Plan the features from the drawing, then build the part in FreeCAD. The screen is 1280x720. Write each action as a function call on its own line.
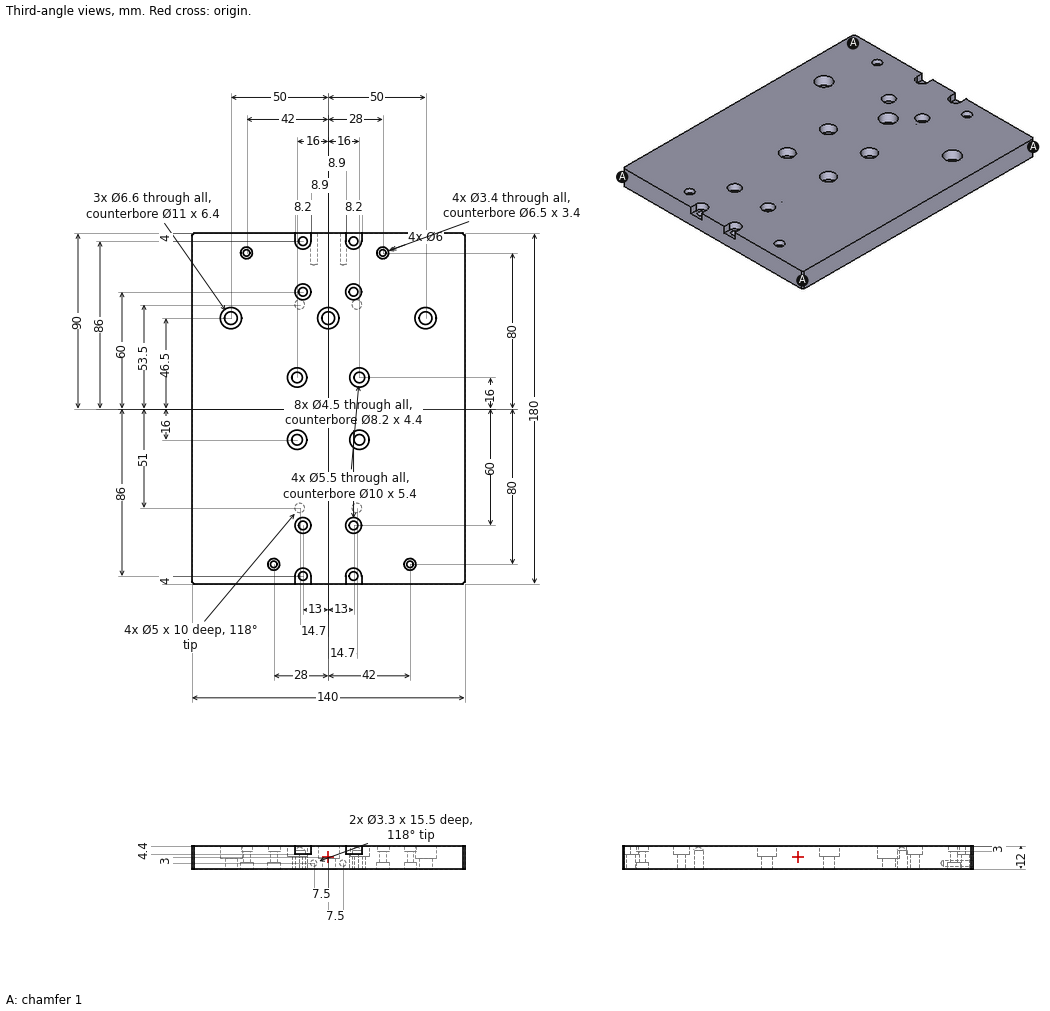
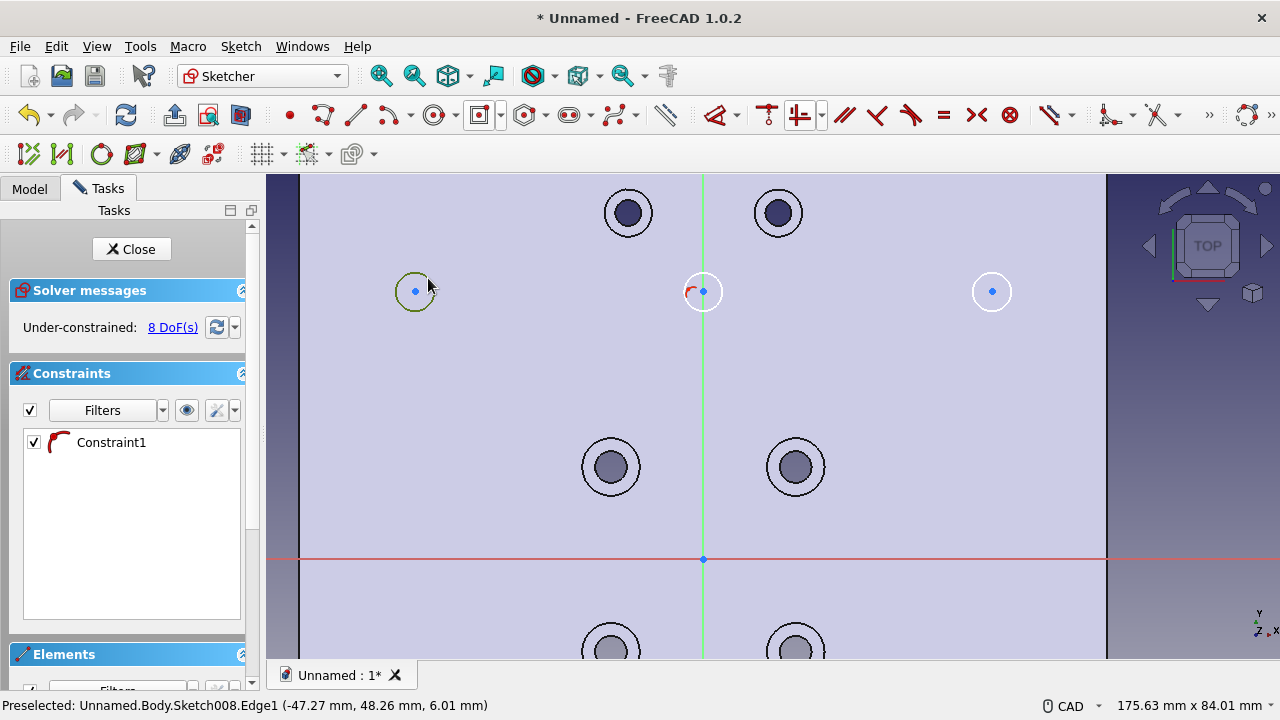
click(717, 279)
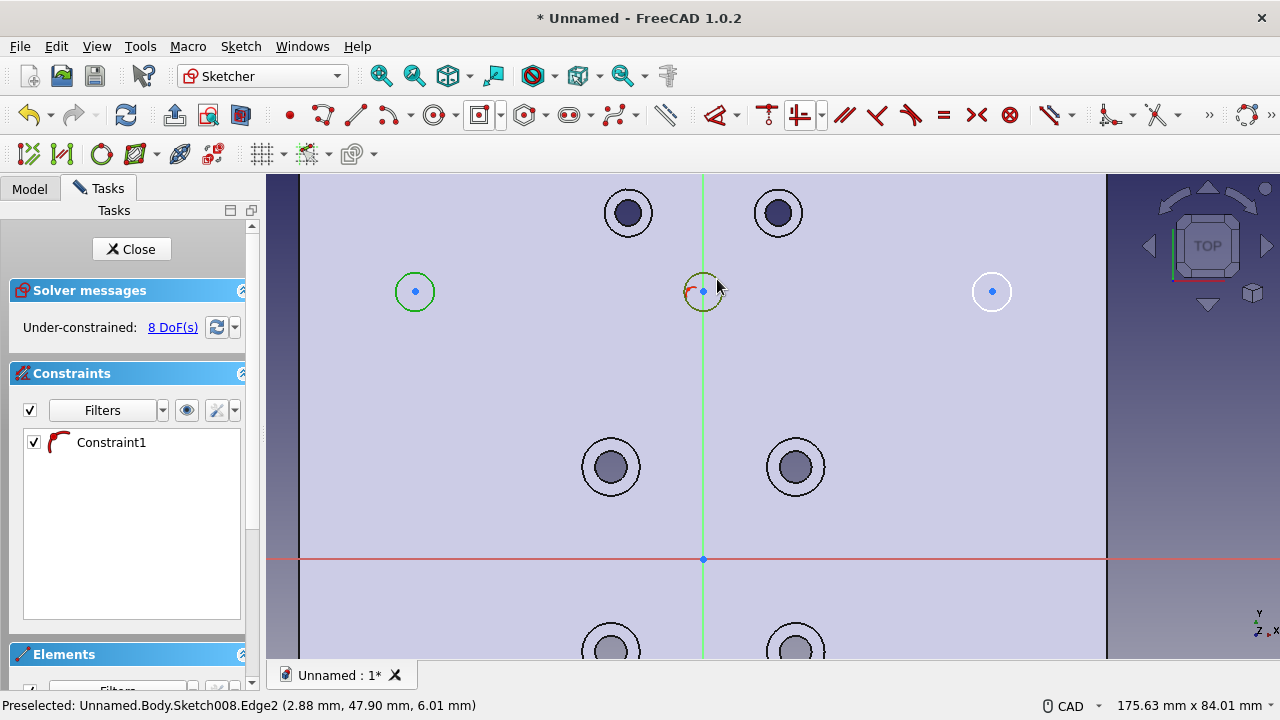
click(1005, 278)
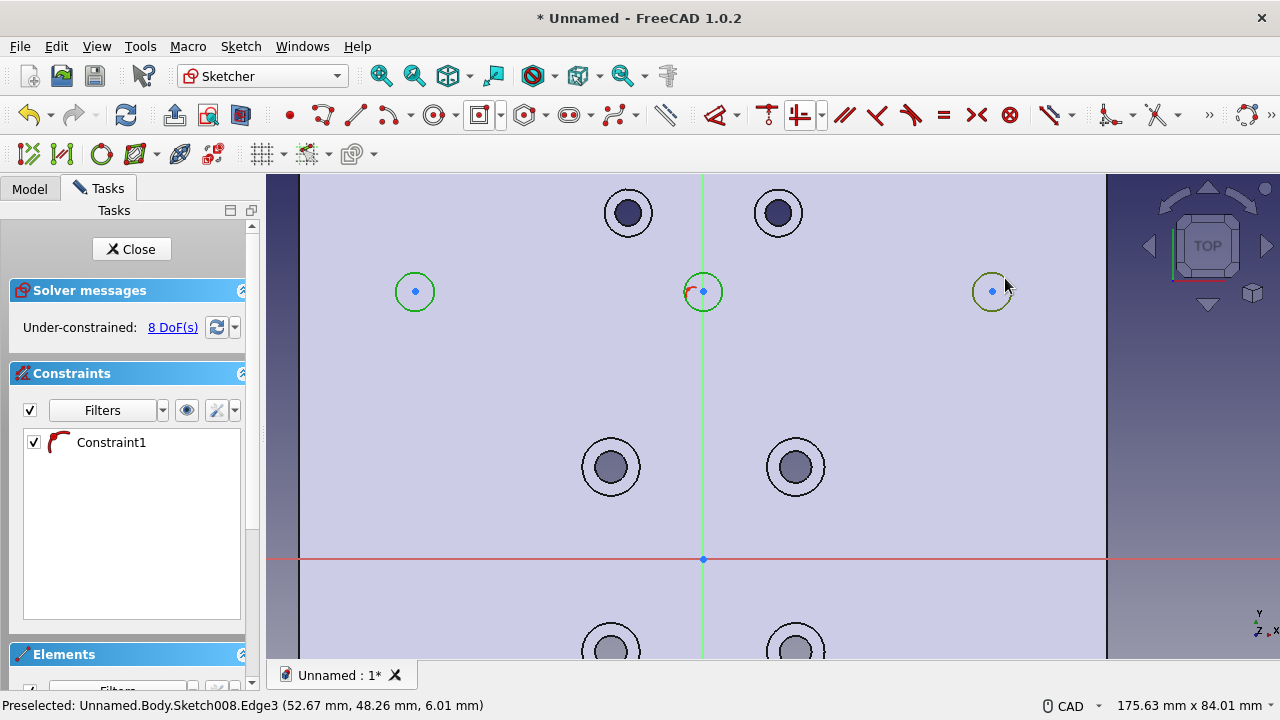
click(944, 116)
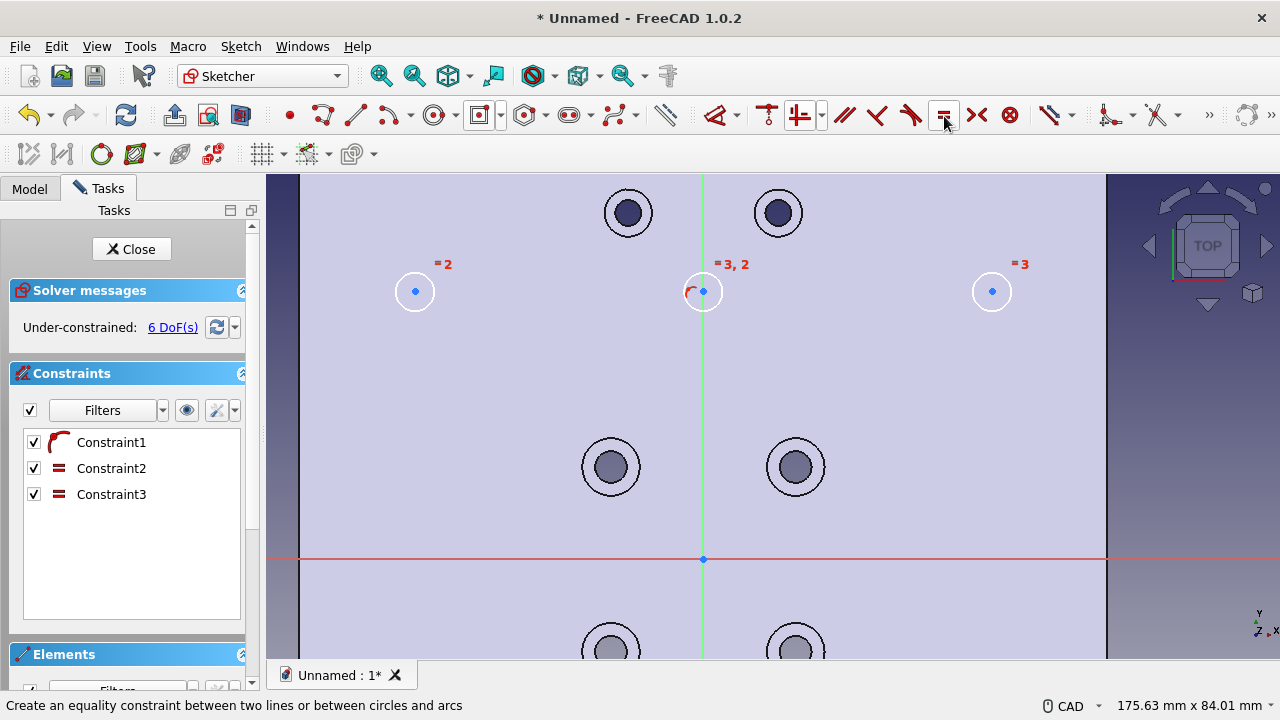
click(714, 116)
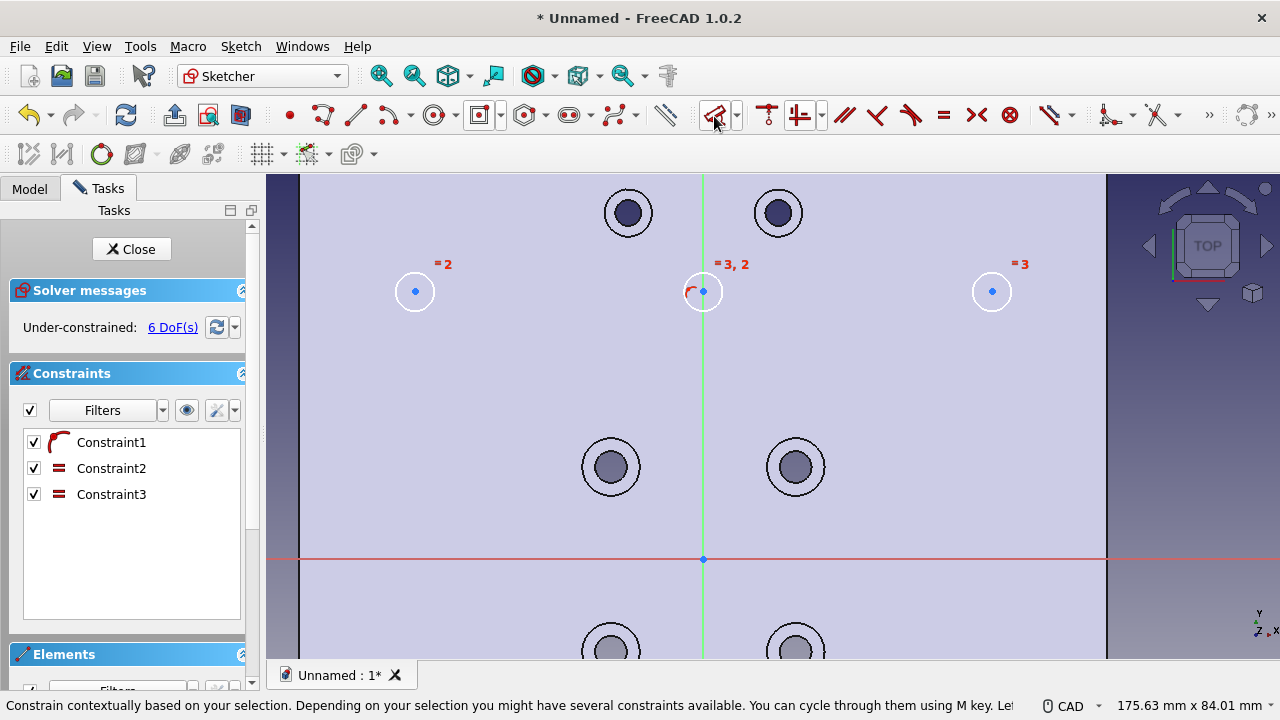
click(428, 278)
click(450, 255)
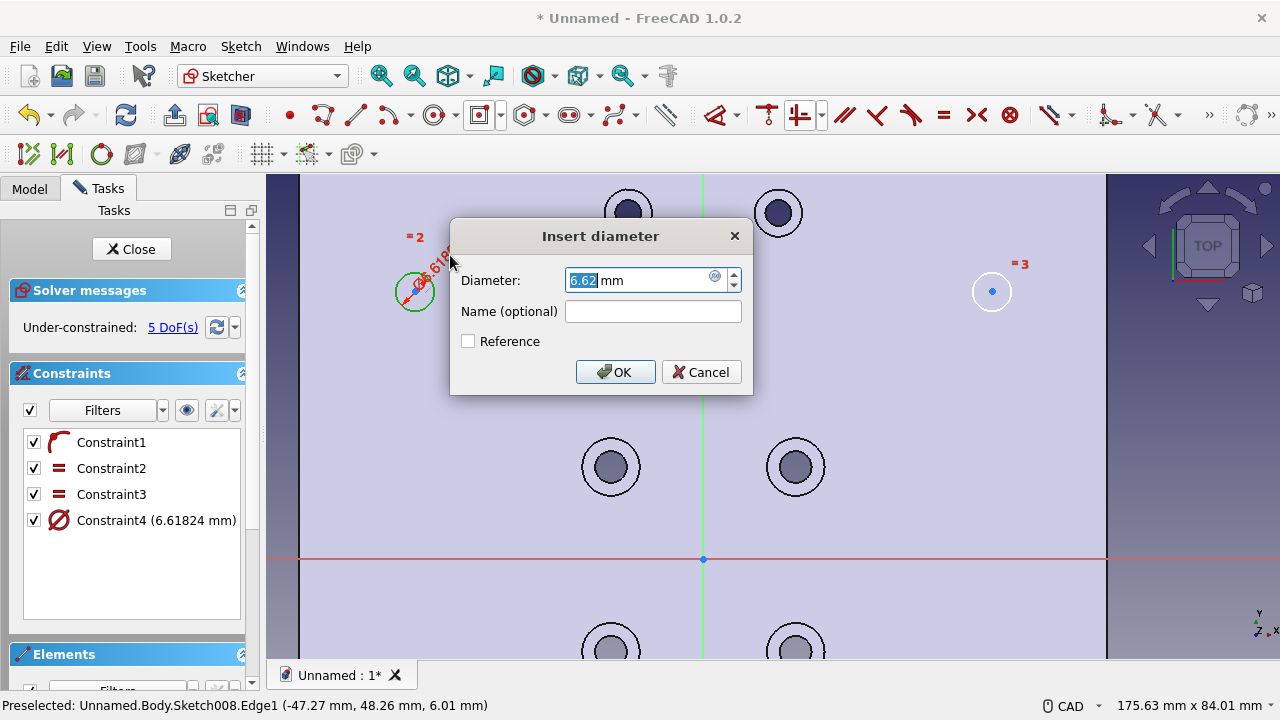
text(6.6)
key(Return)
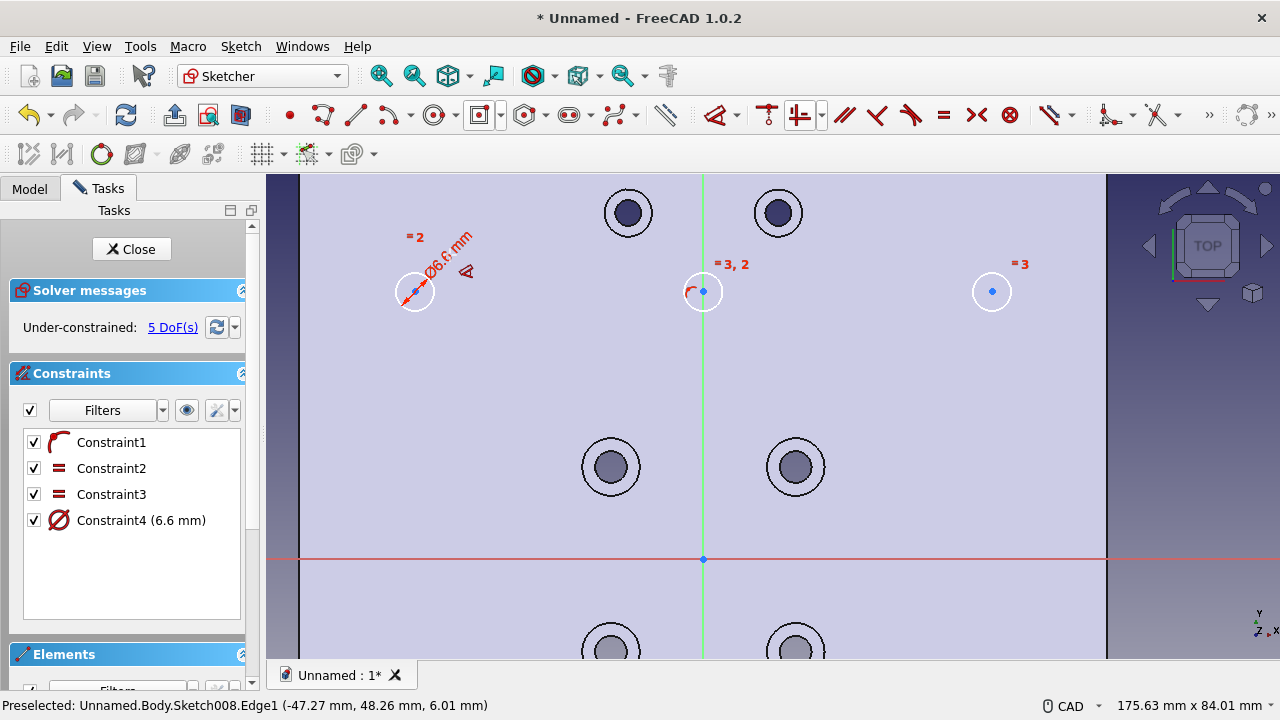
click(415, 292)
click(559, 593)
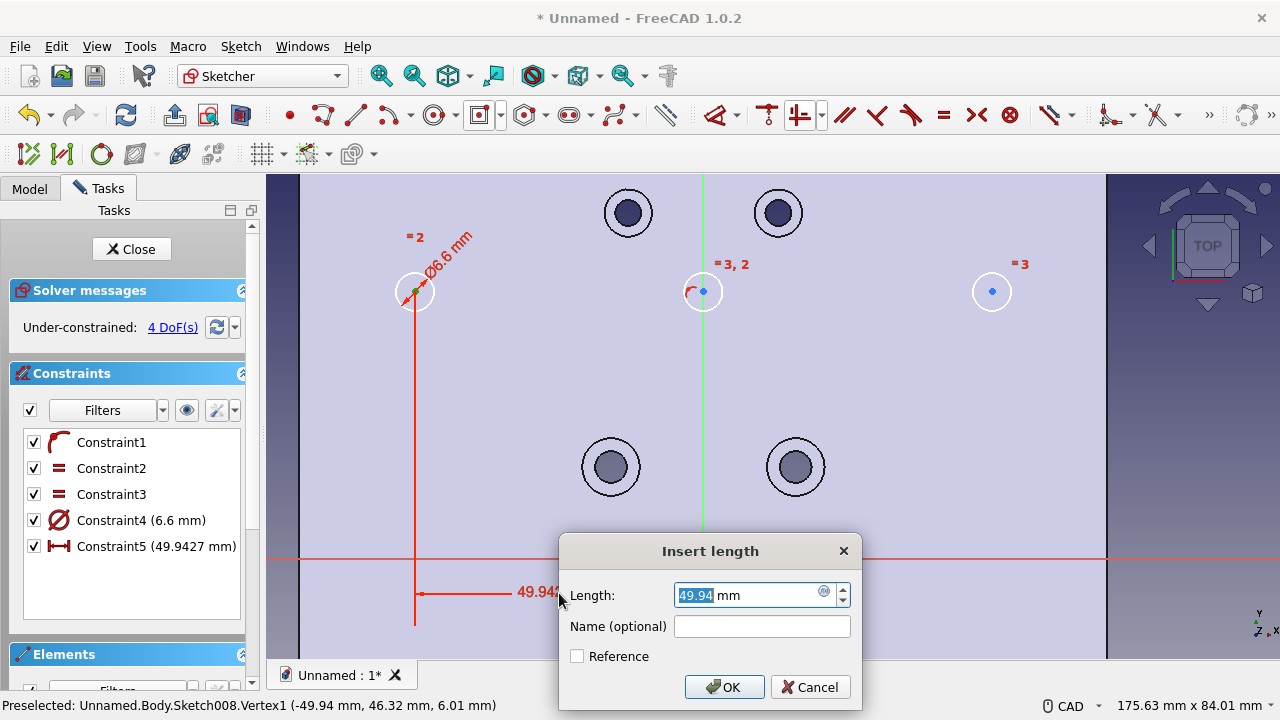
text(50)
key(Return)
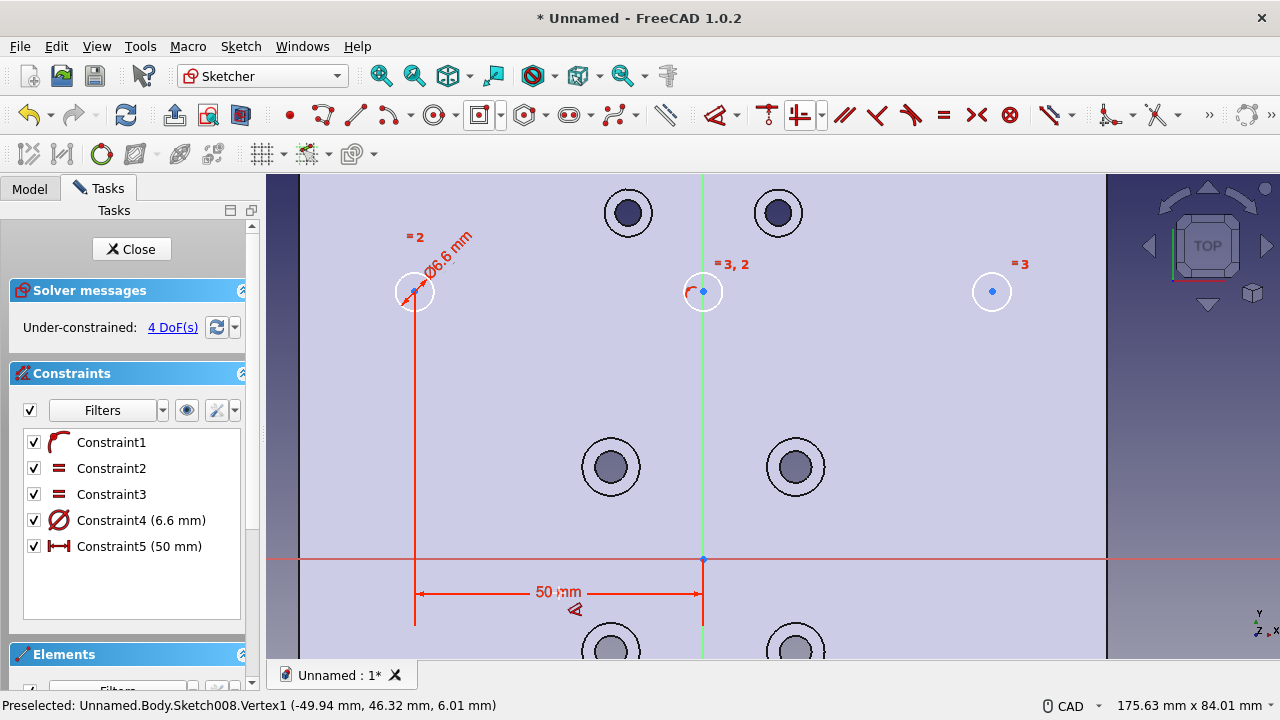
click(992, 292)
click(848, 593)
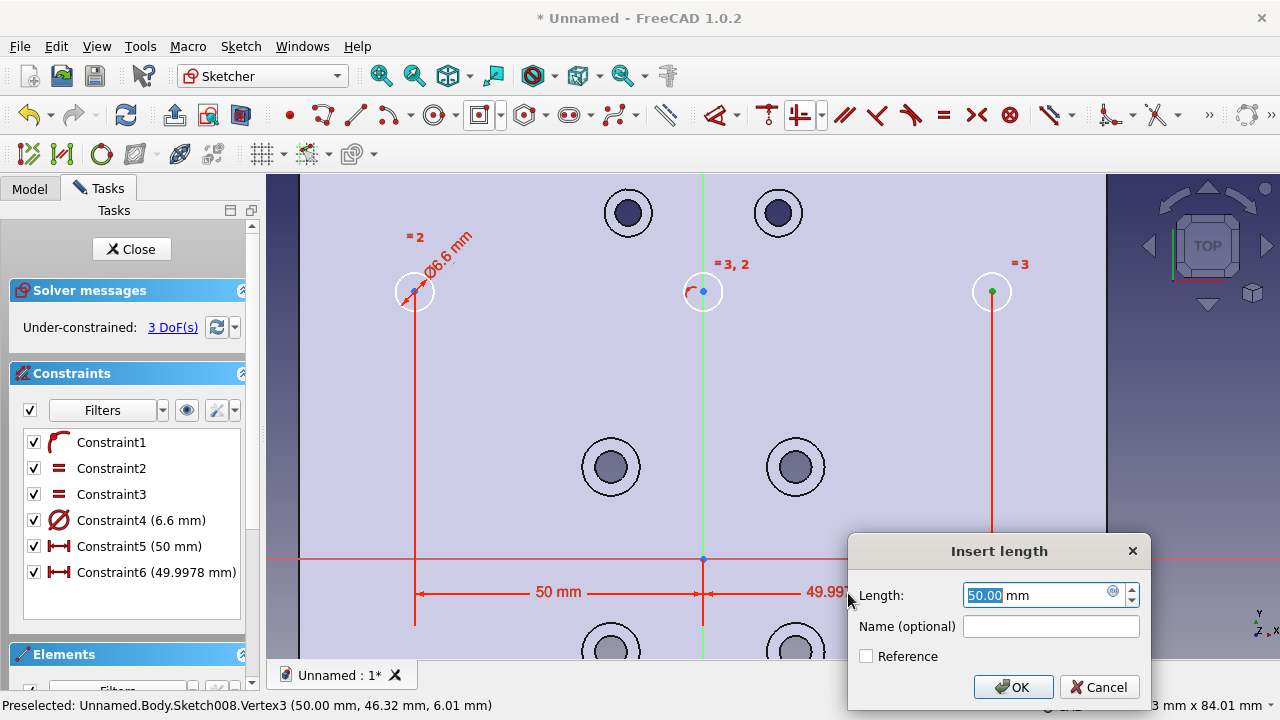
text(50)
key(Return)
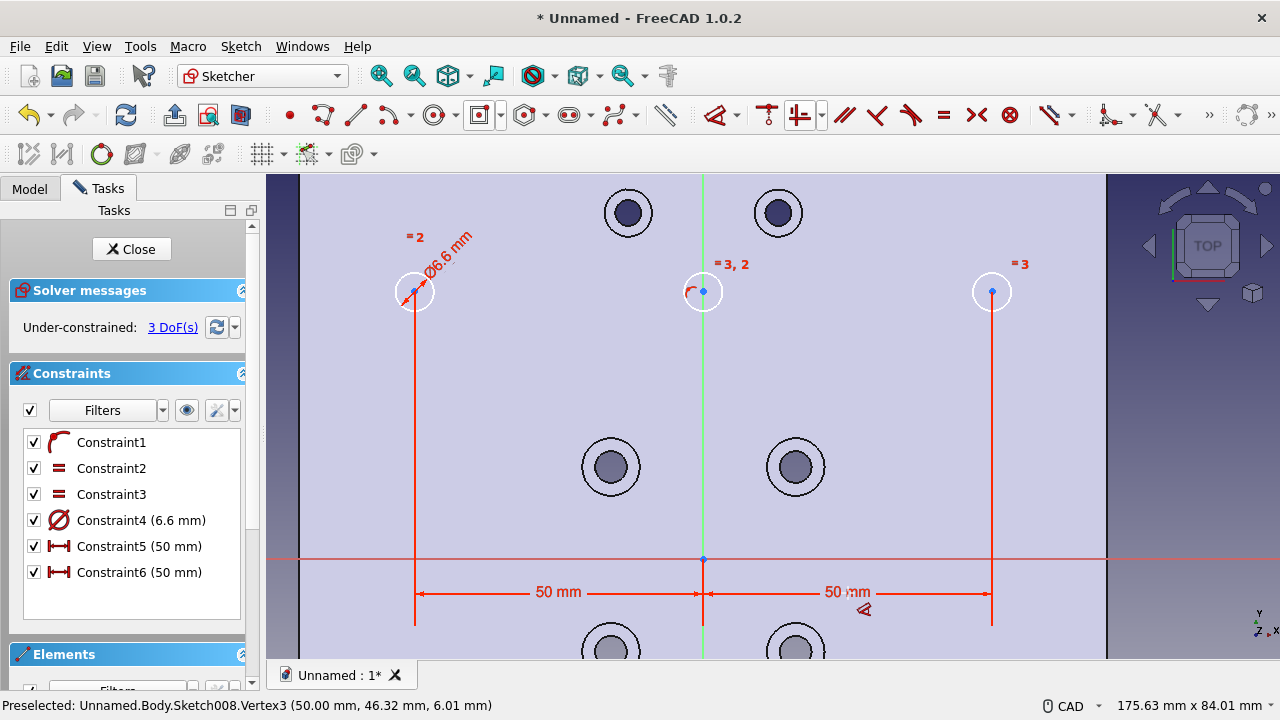
click(415, 292)
click(381, 426)